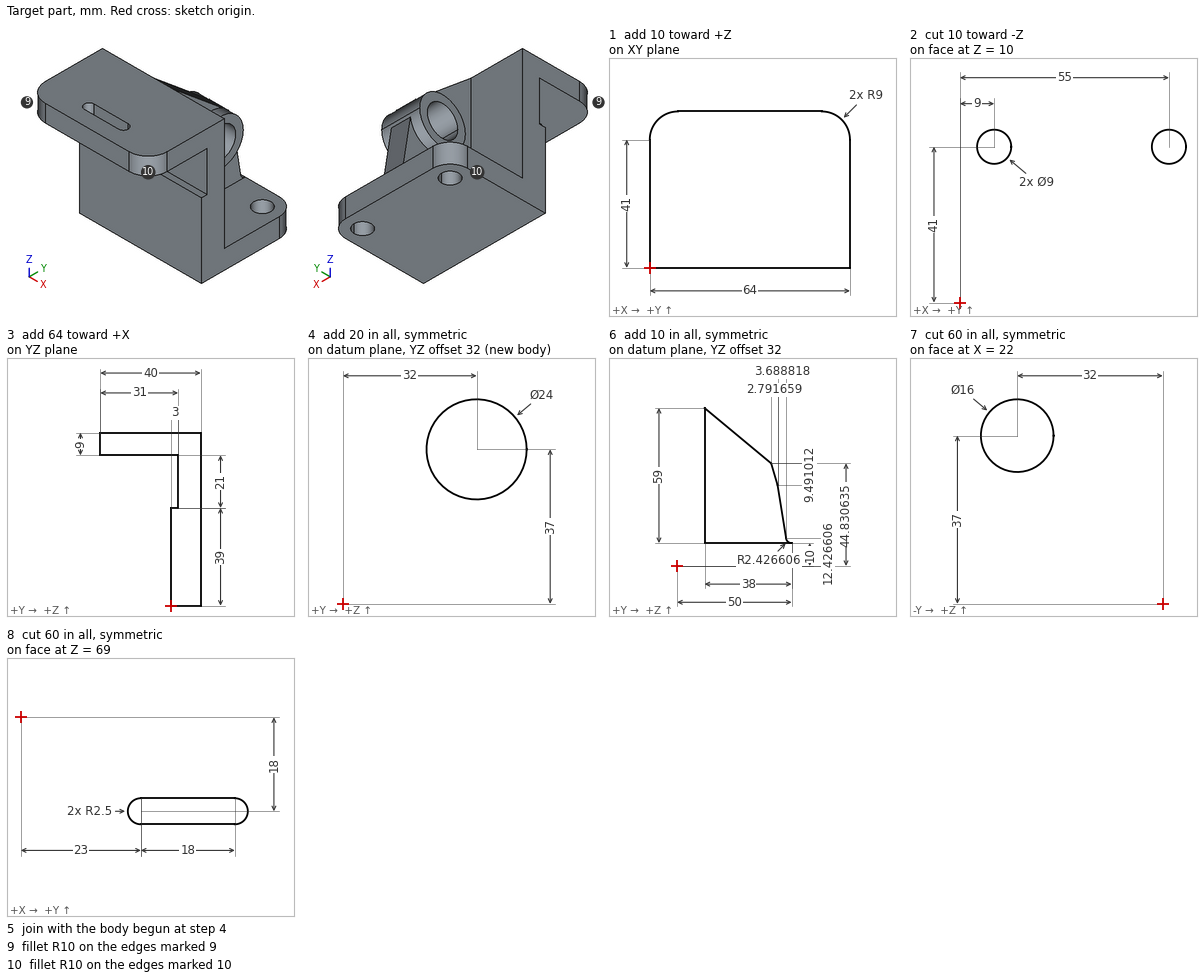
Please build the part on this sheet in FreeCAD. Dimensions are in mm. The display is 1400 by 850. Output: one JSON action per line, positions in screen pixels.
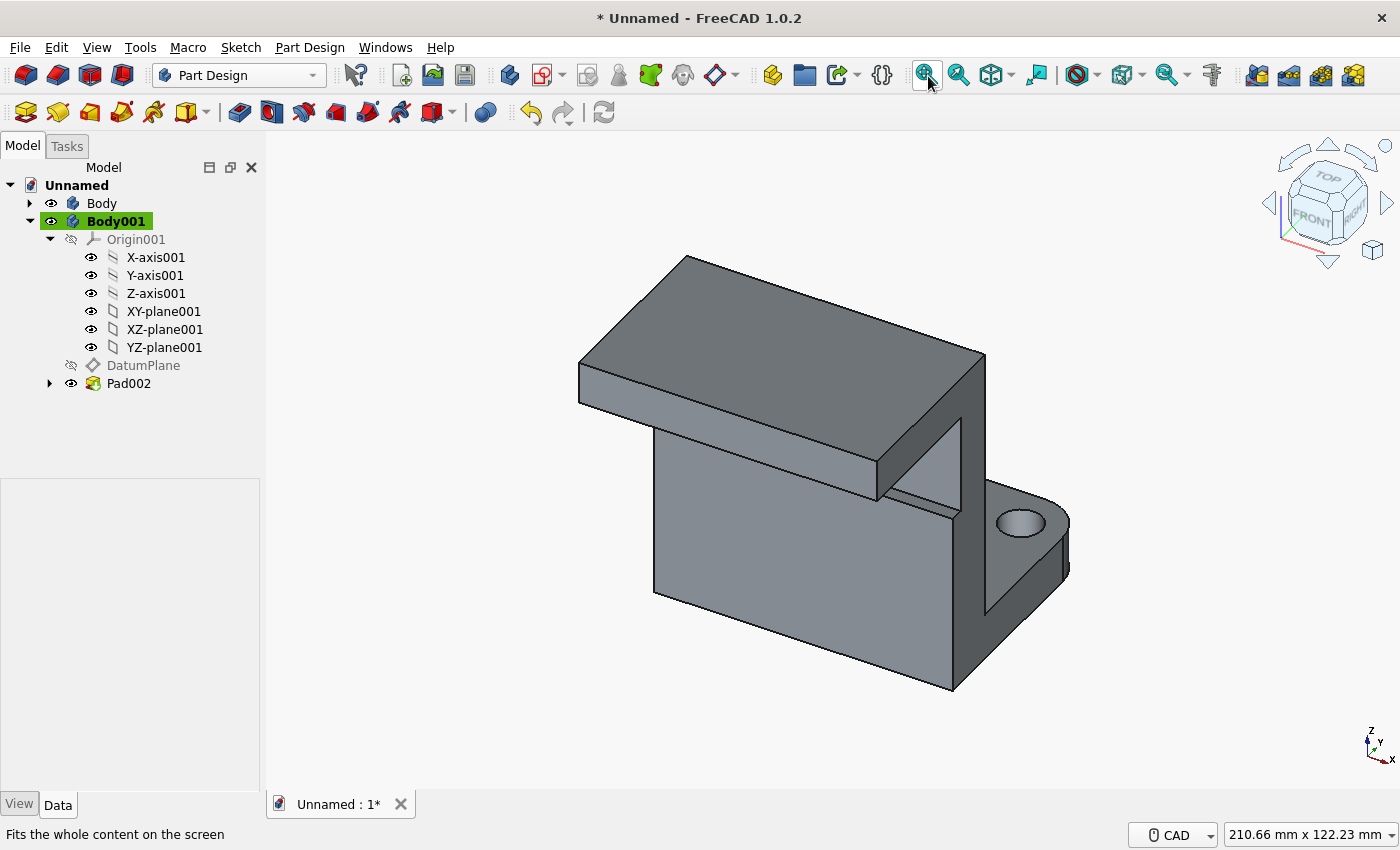
{"action": "double_click", "coordinate": [96, 203]}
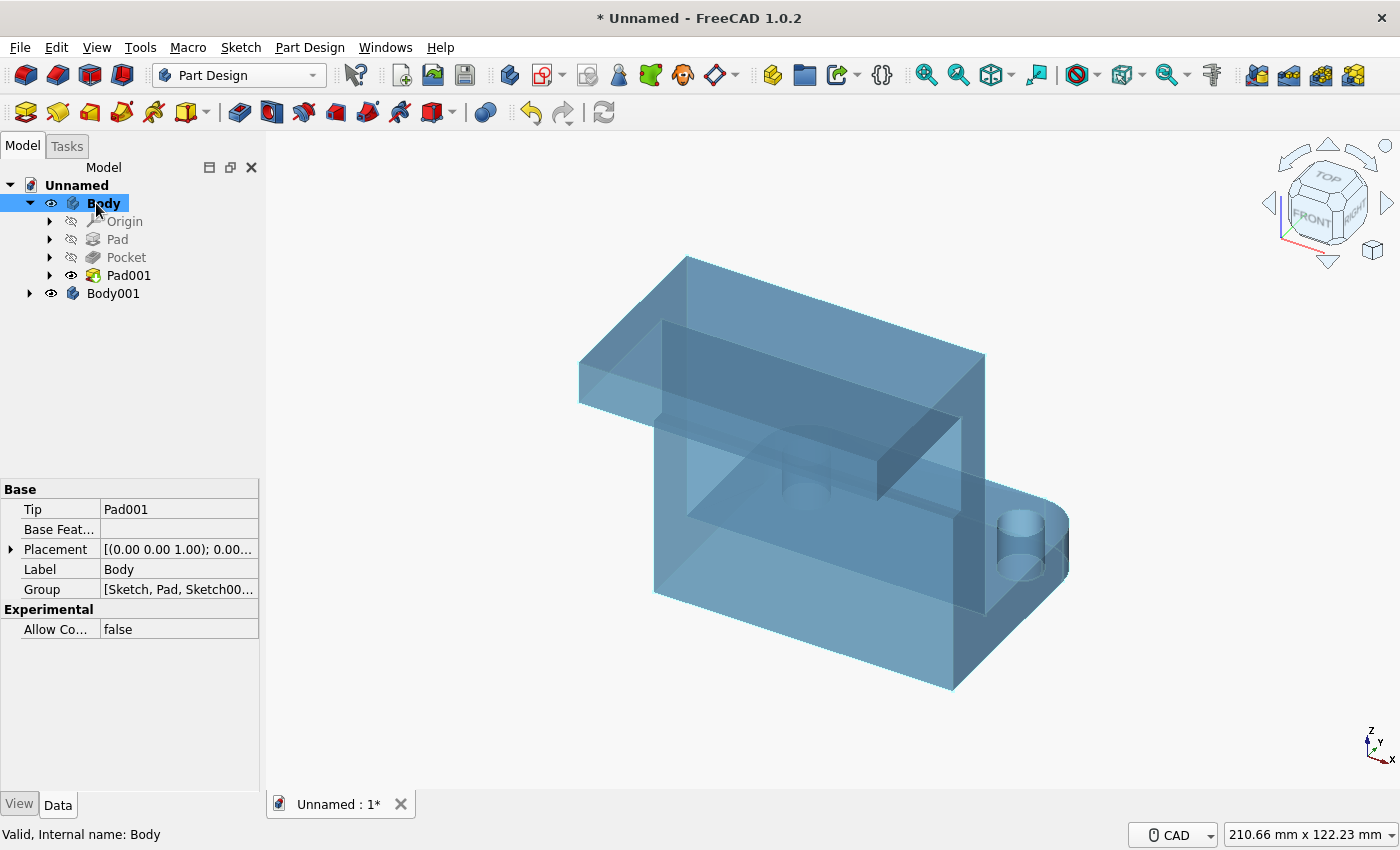
{"action": "left_click", "coordinate": [96, 203]}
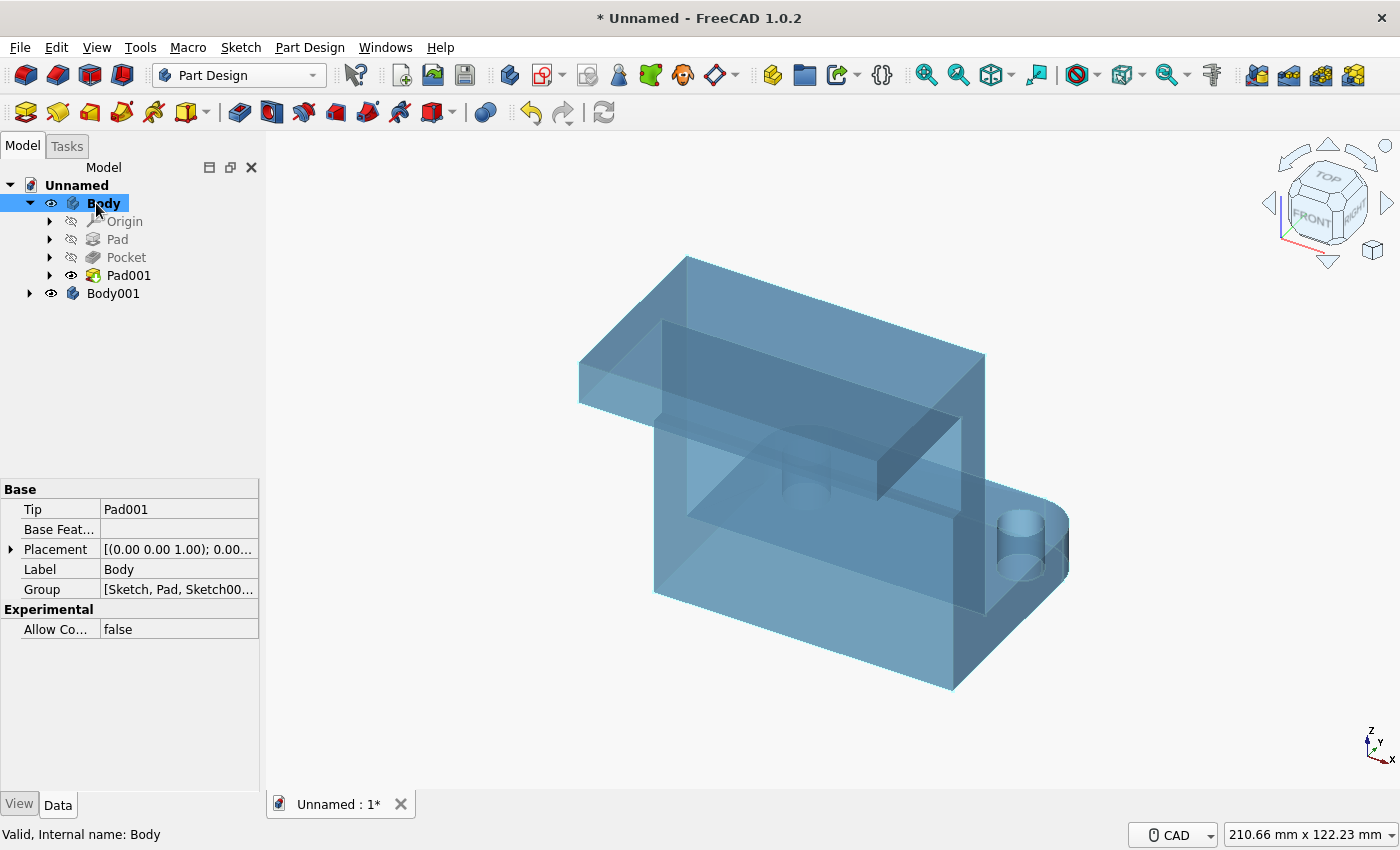
{"action": "left_click", "coordinate": [146, 629]}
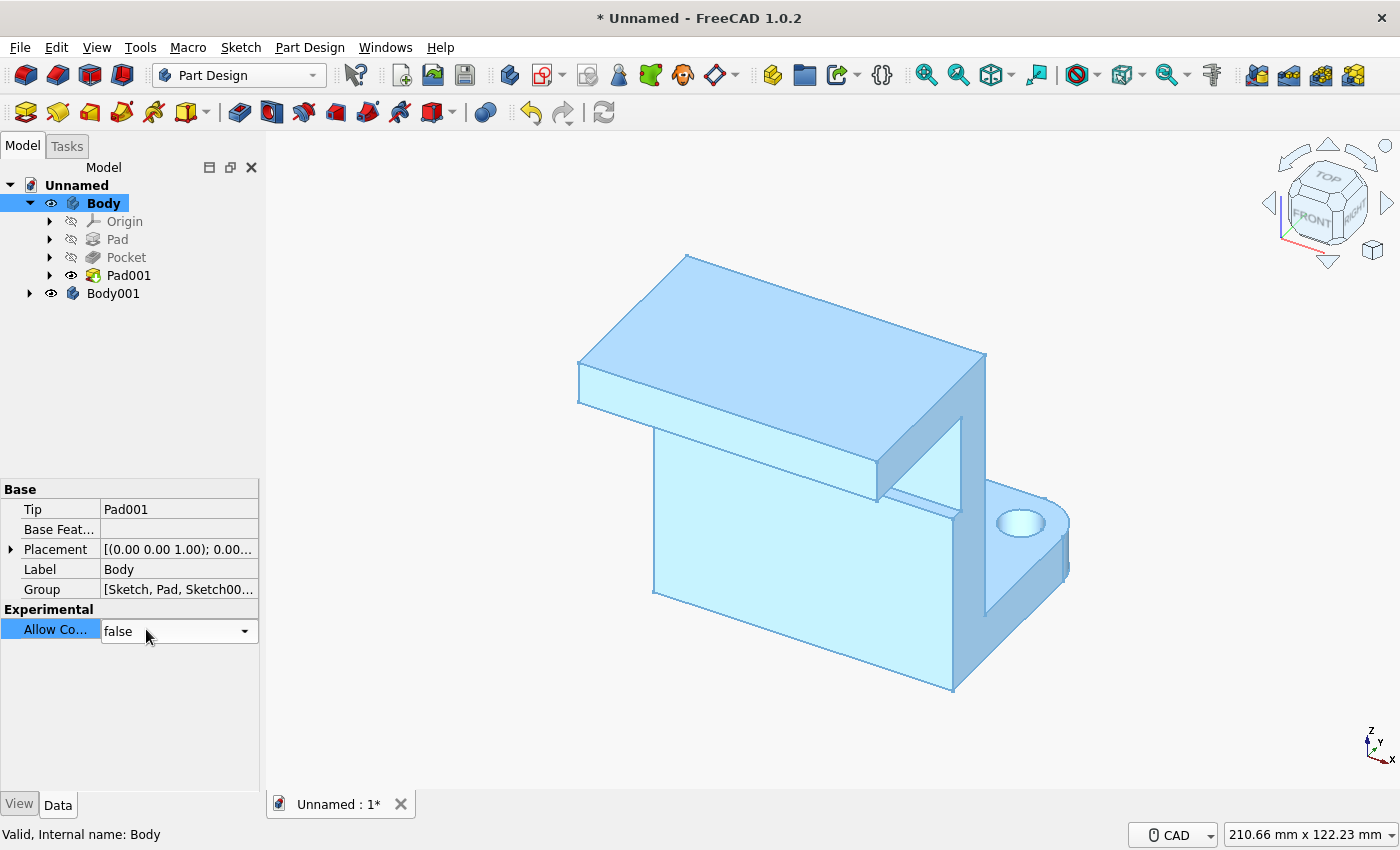
{"action": "left_click", "coordinate": [146, 629]}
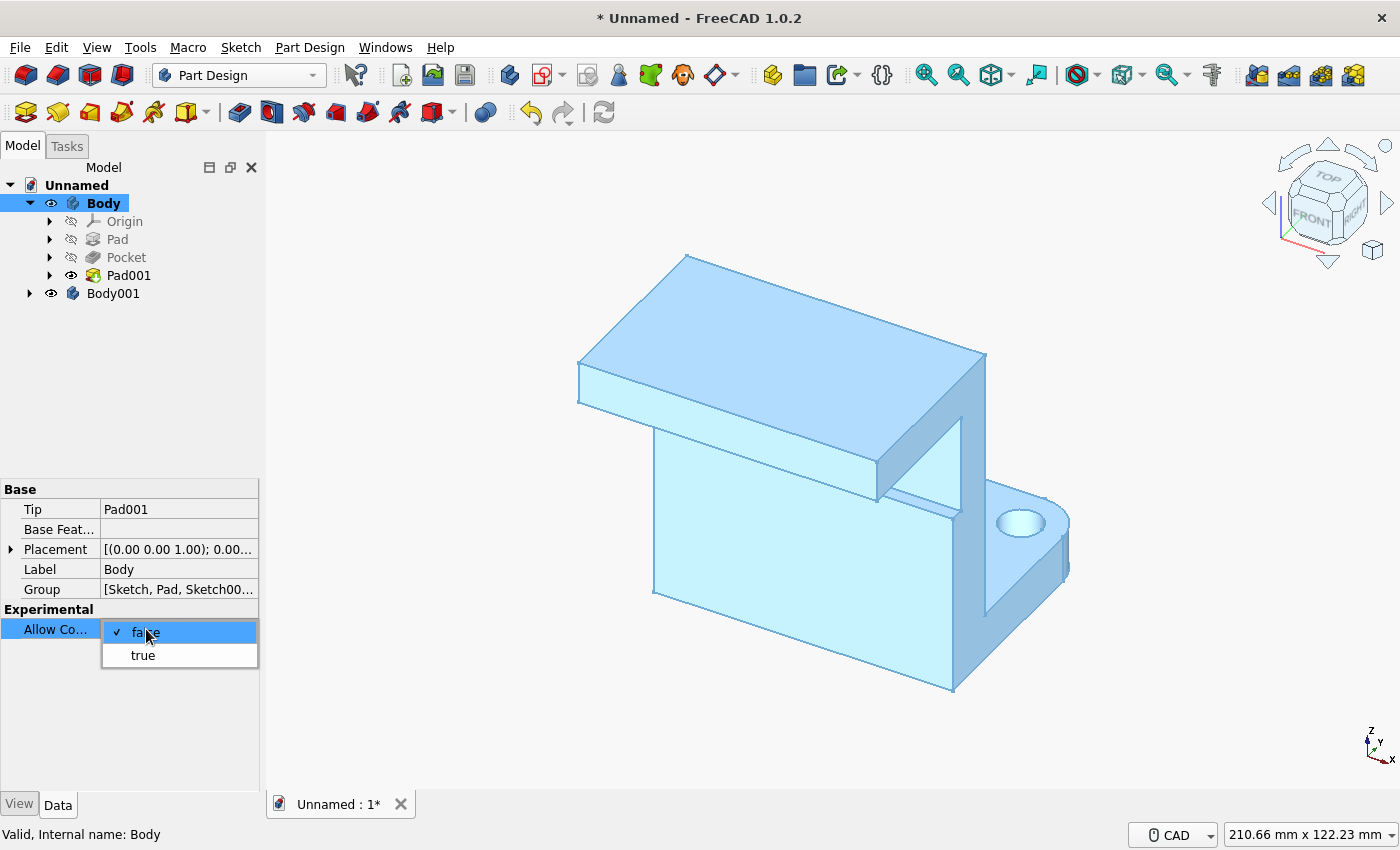
{"action": "left_click", "coordinate": [179, 656]}
{"action": "key", "text": "Return"}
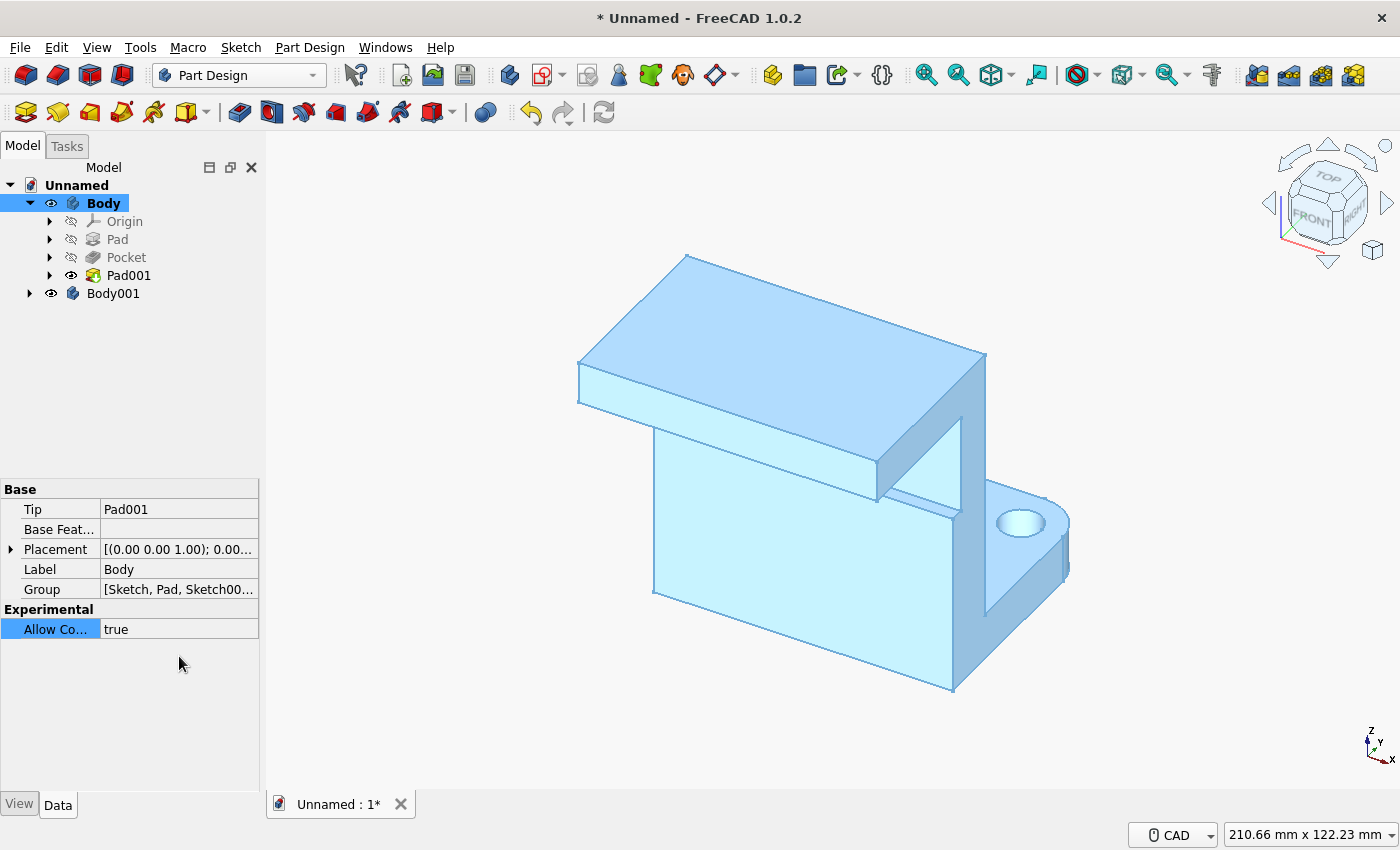
{"action": "left_click", "coordinate": [96, 293]}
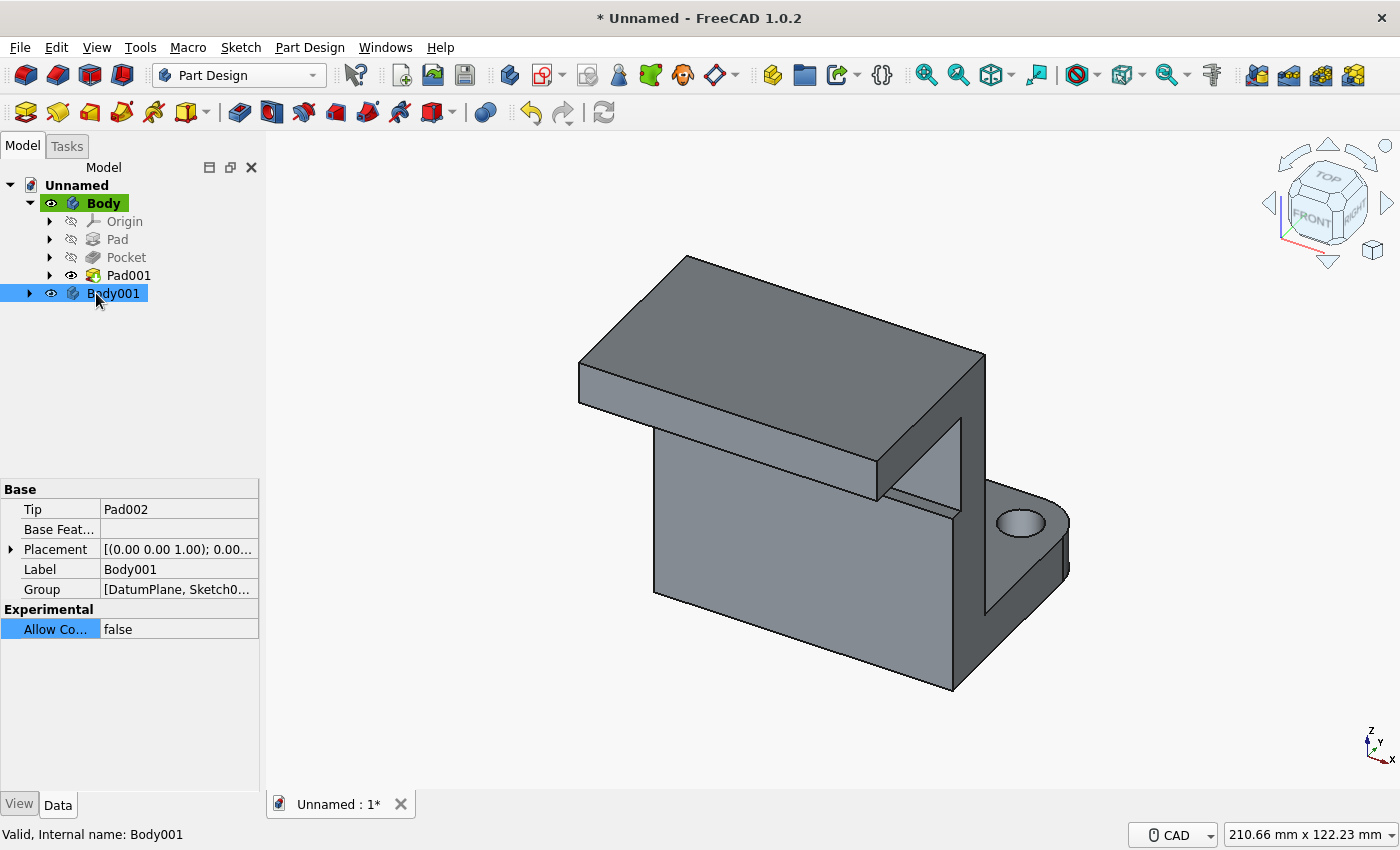
{"action": "left_click", "coordinate": [486, 112]}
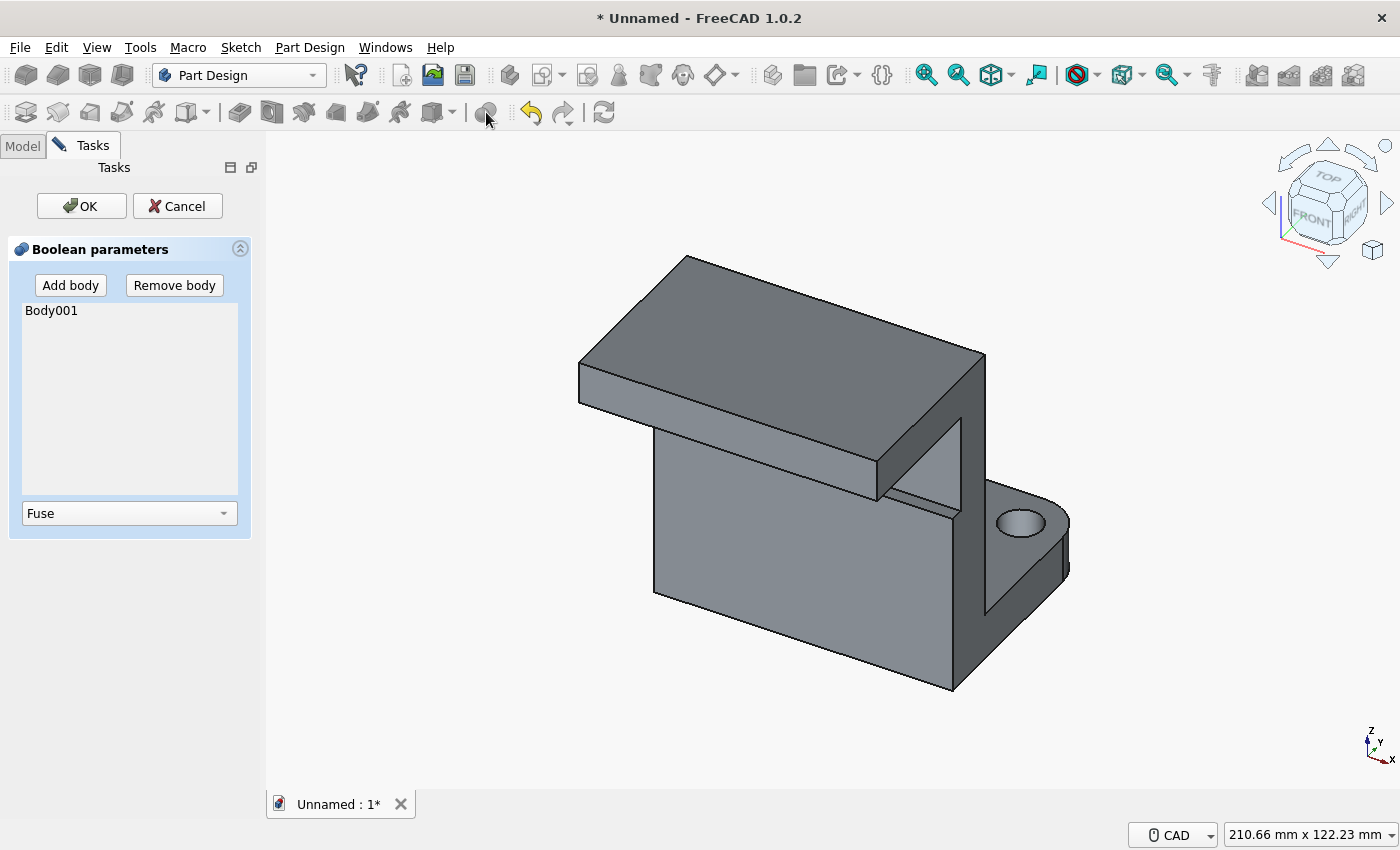
{"action": "left_click", "coordinate": [82, 206]}